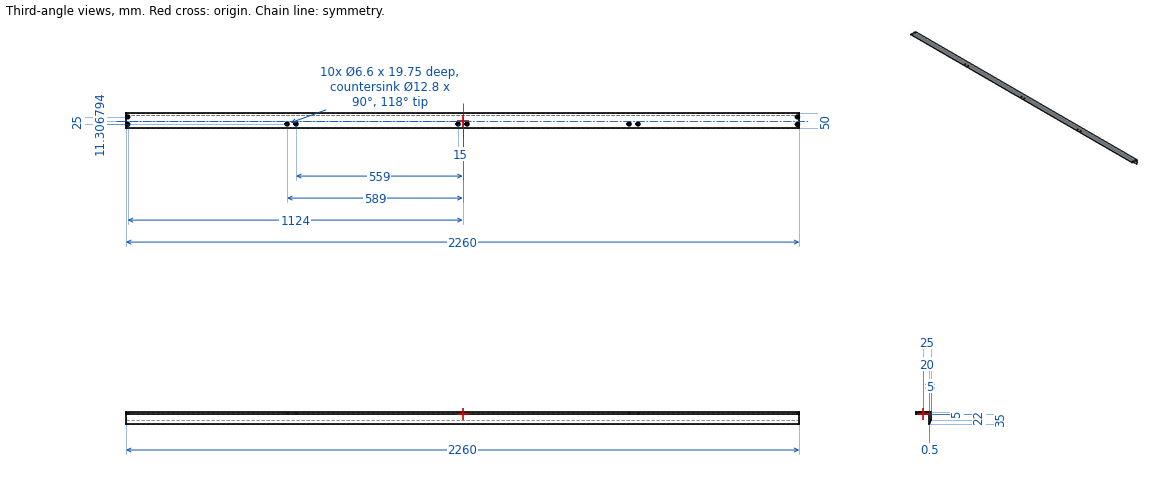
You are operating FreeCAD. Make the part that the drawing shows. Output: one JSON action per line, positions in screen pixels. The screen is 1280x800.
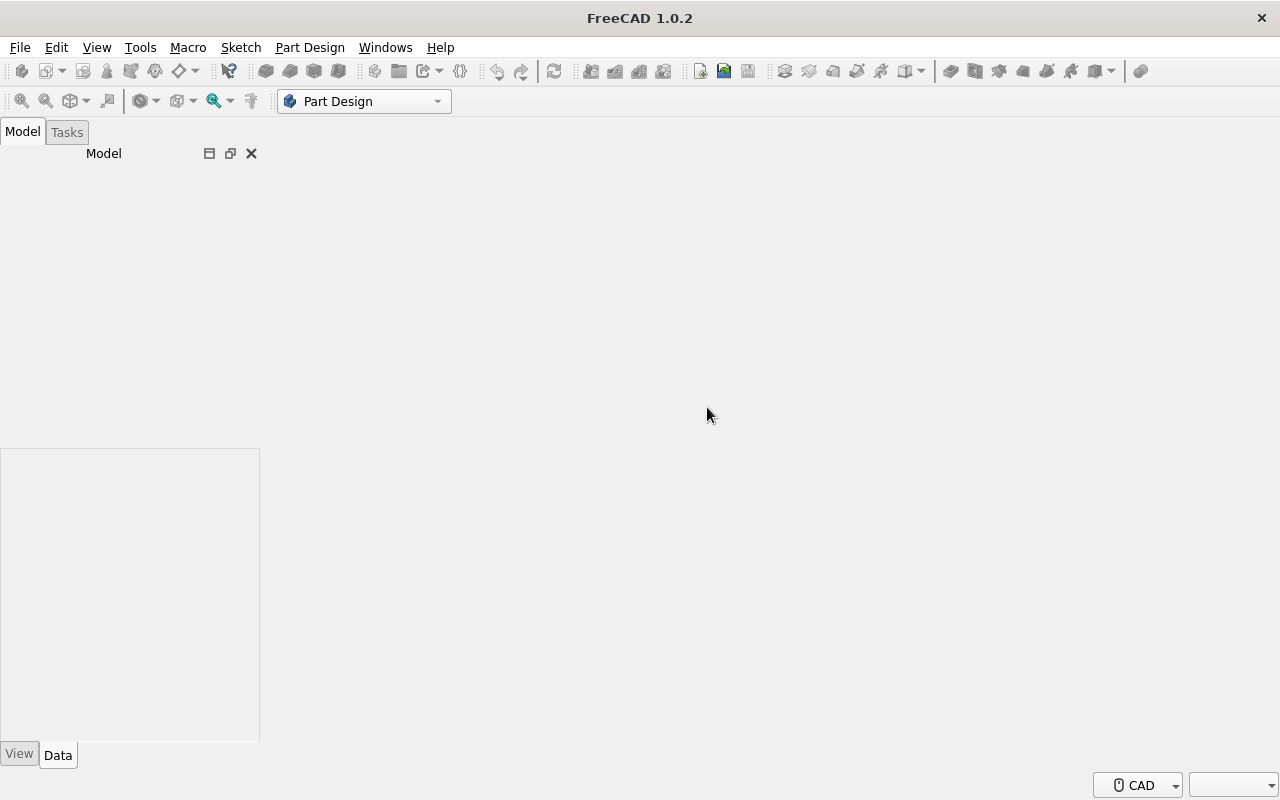
{"action": "left_click", "coordinate": [700, 72]}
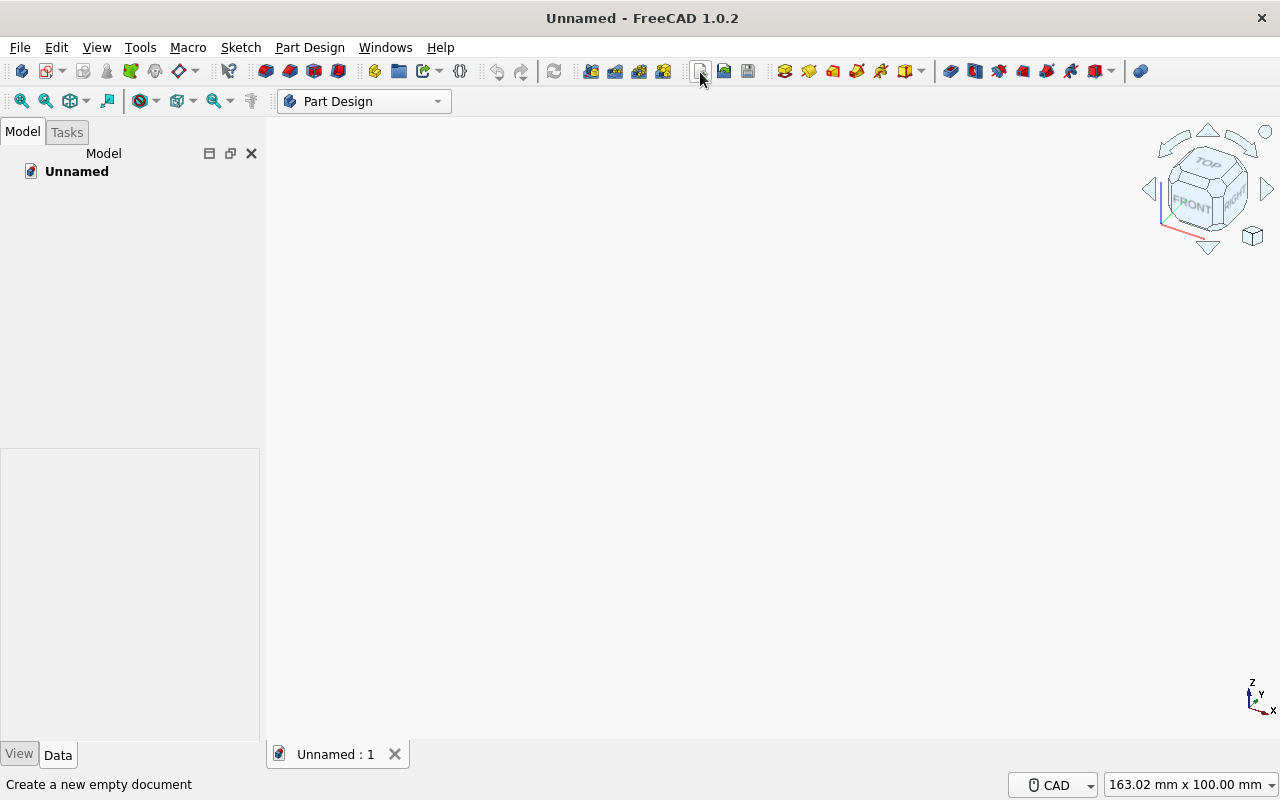
{"action": "left_click", "coordinate": [46, 72]}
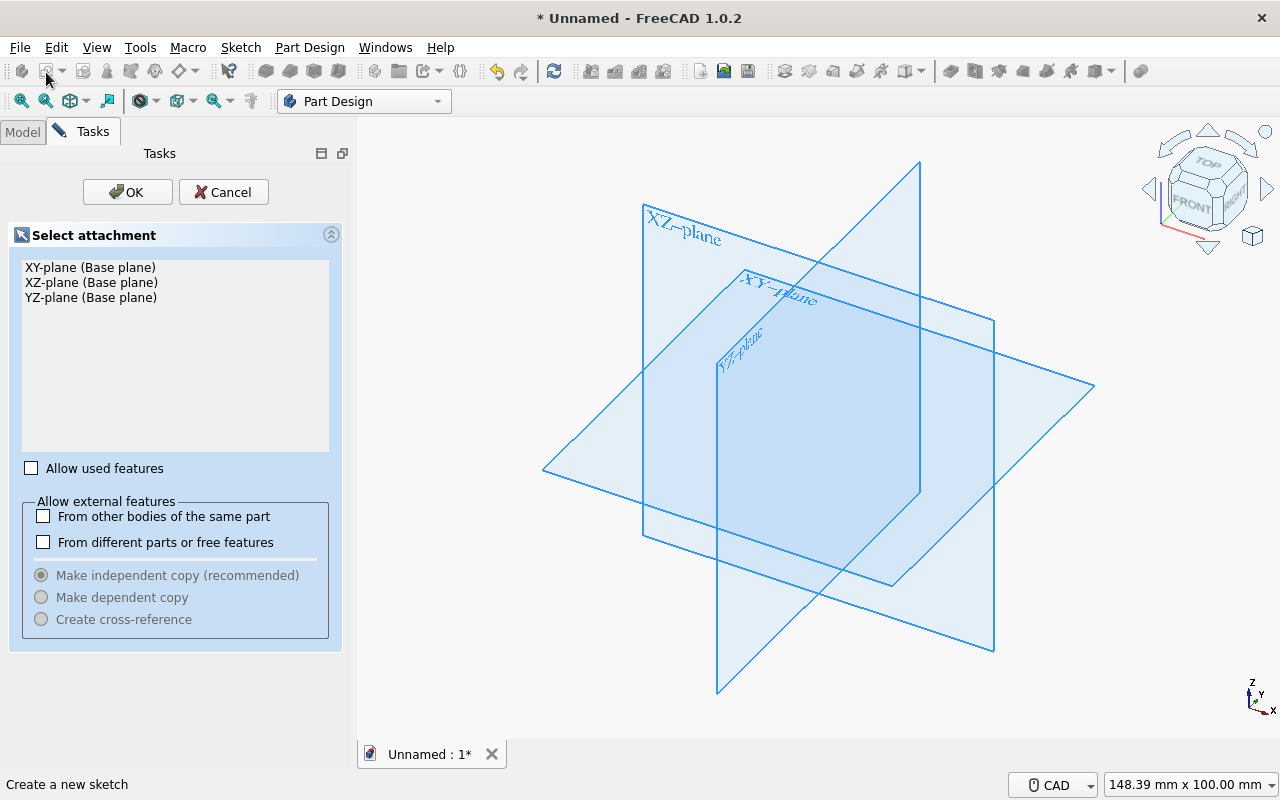
{"action": "left_click", "coordinate": [82, 268]}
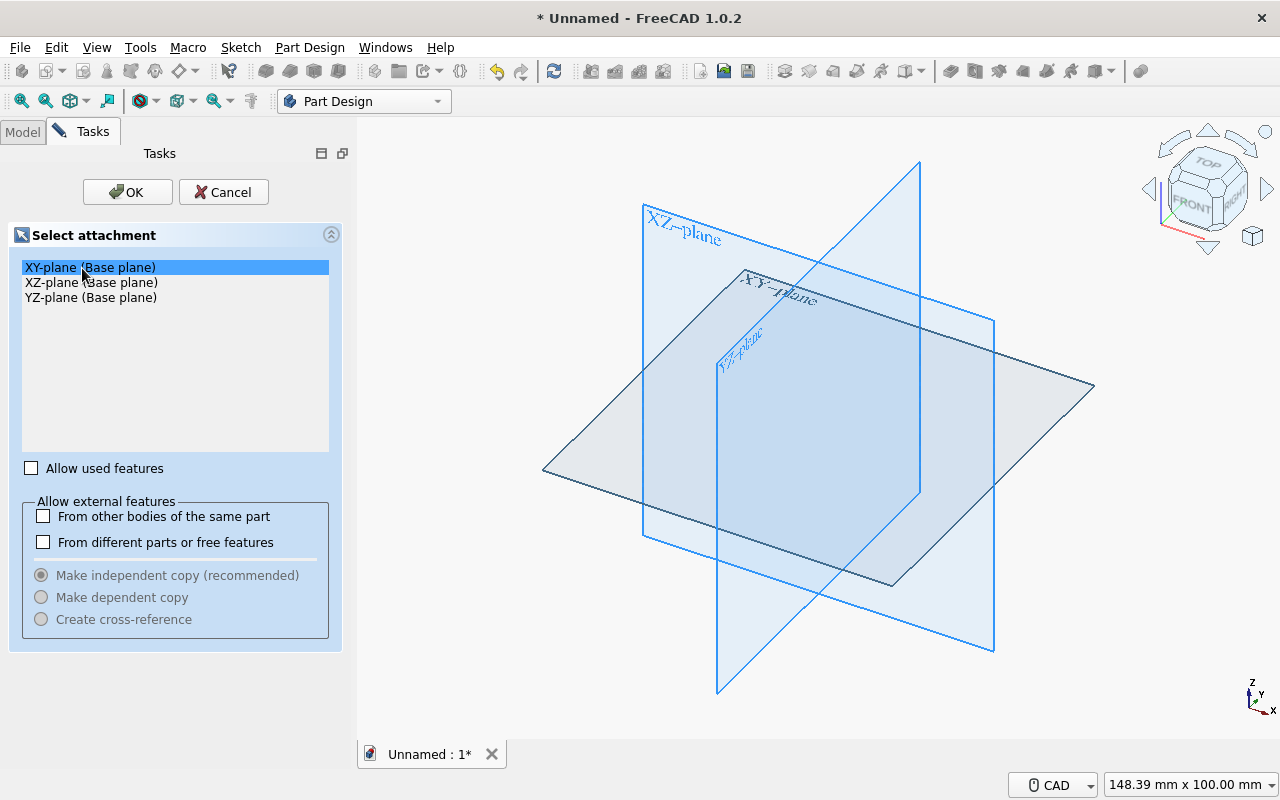
{"action": "left_click", "coordinate": [128, 192]}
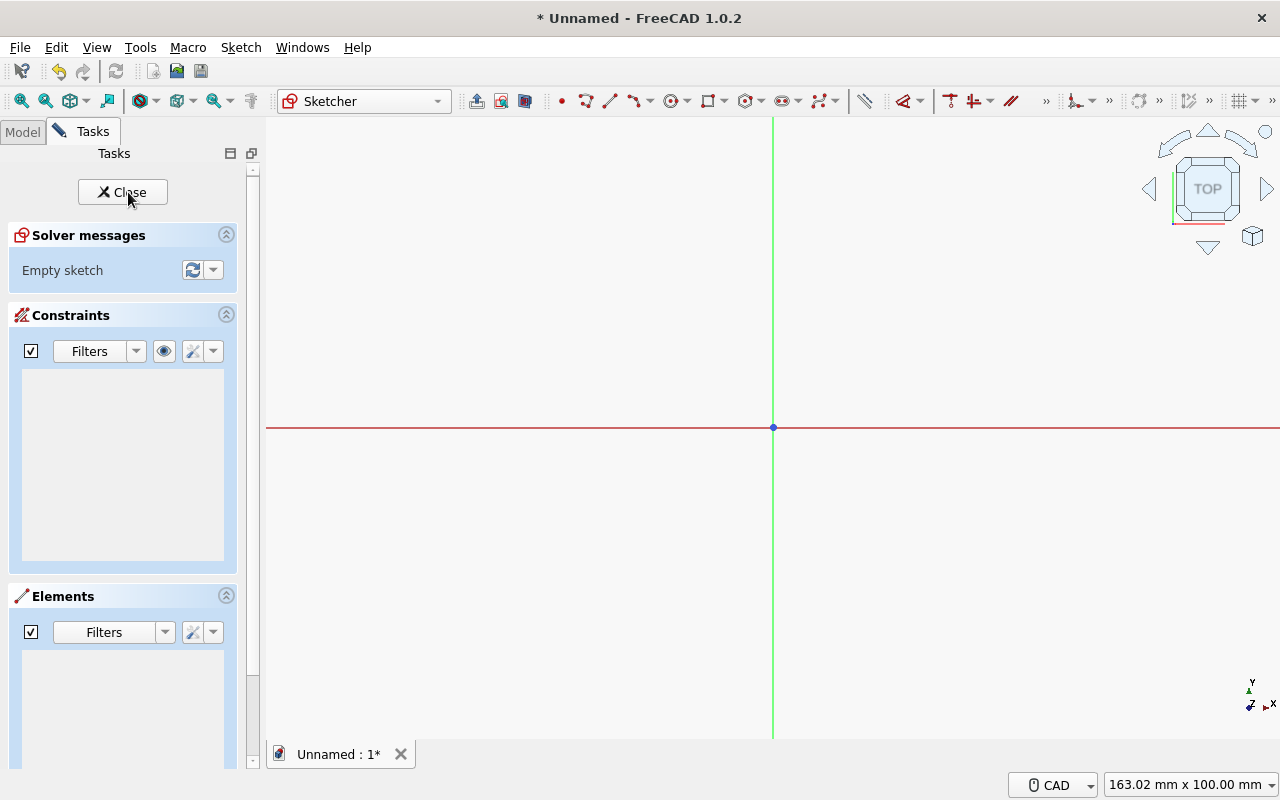
{"action": "scroll", "coordinate": [701, 428], "scroll_direction": "down", "scroll_amount": 15}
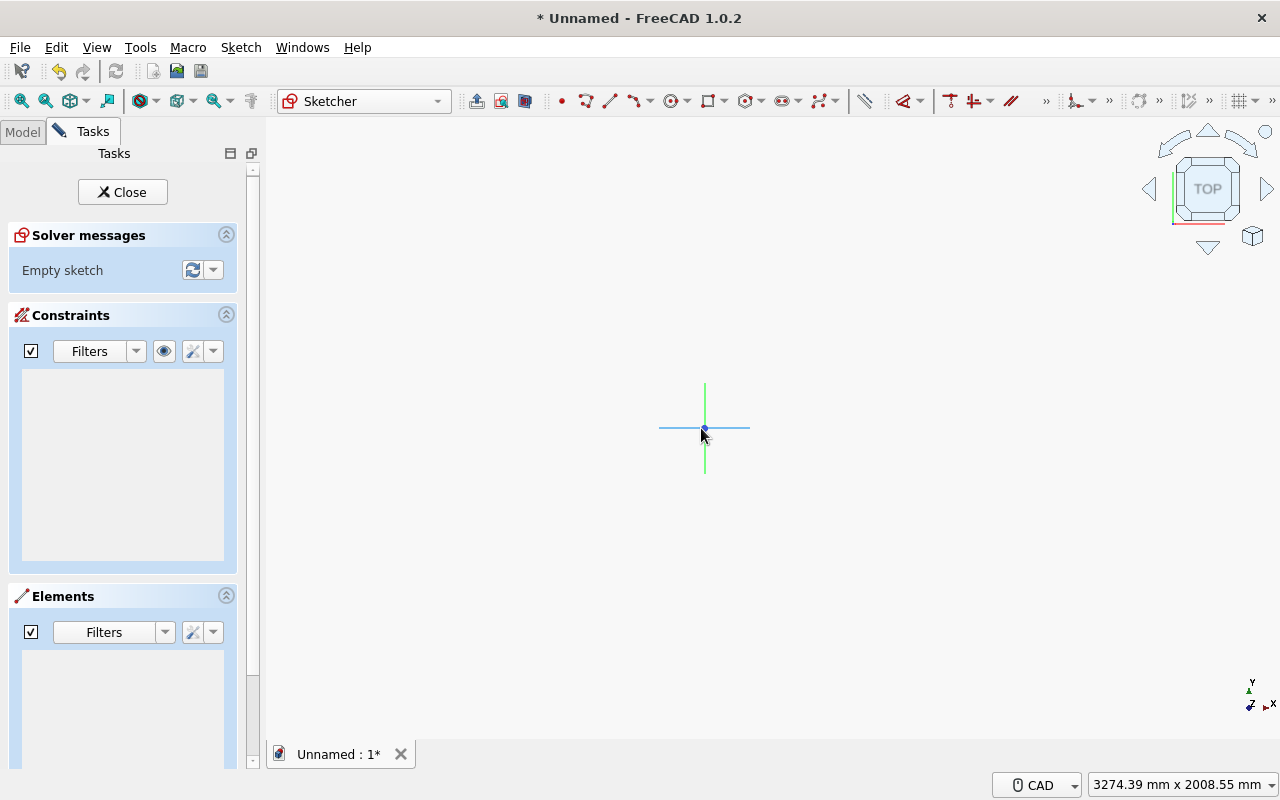
{"action": "left_click", "coordinate": [726, 102]}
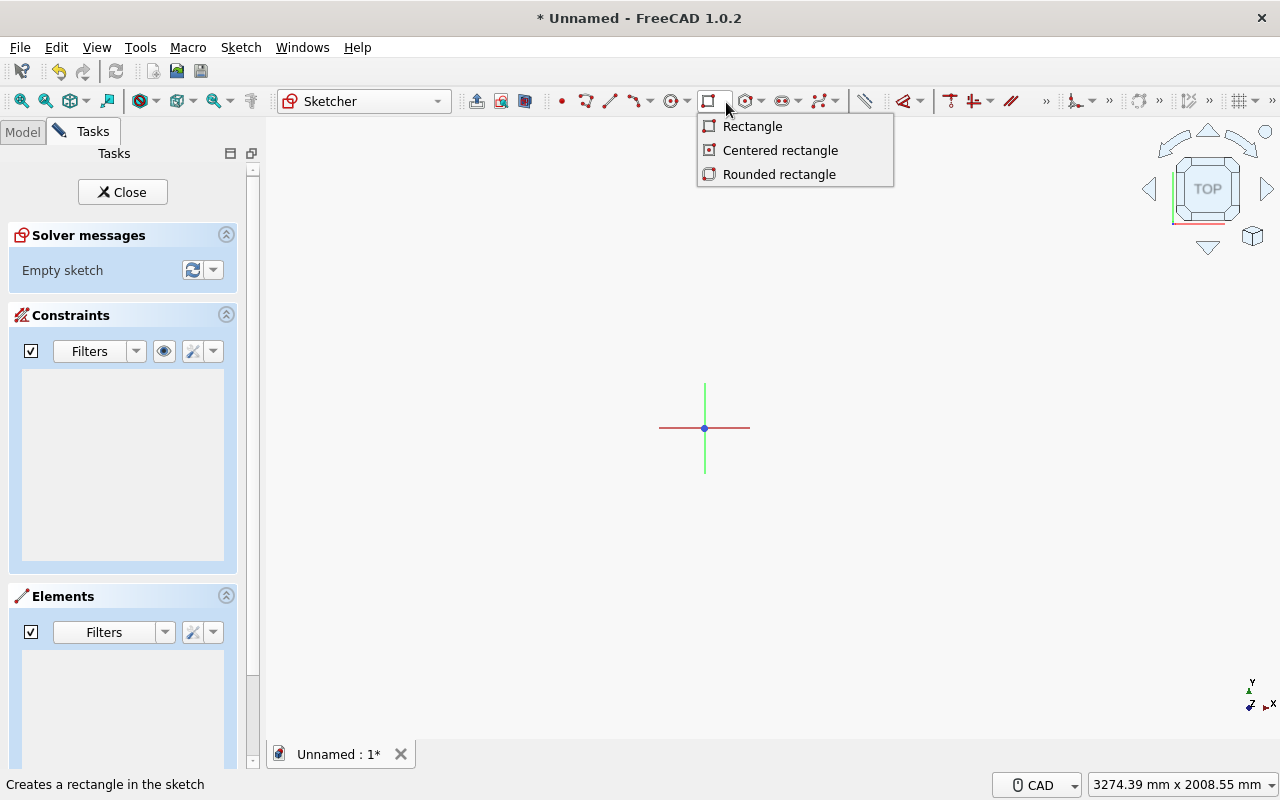
{"action": "left_click", "coordinate": [796, 150]}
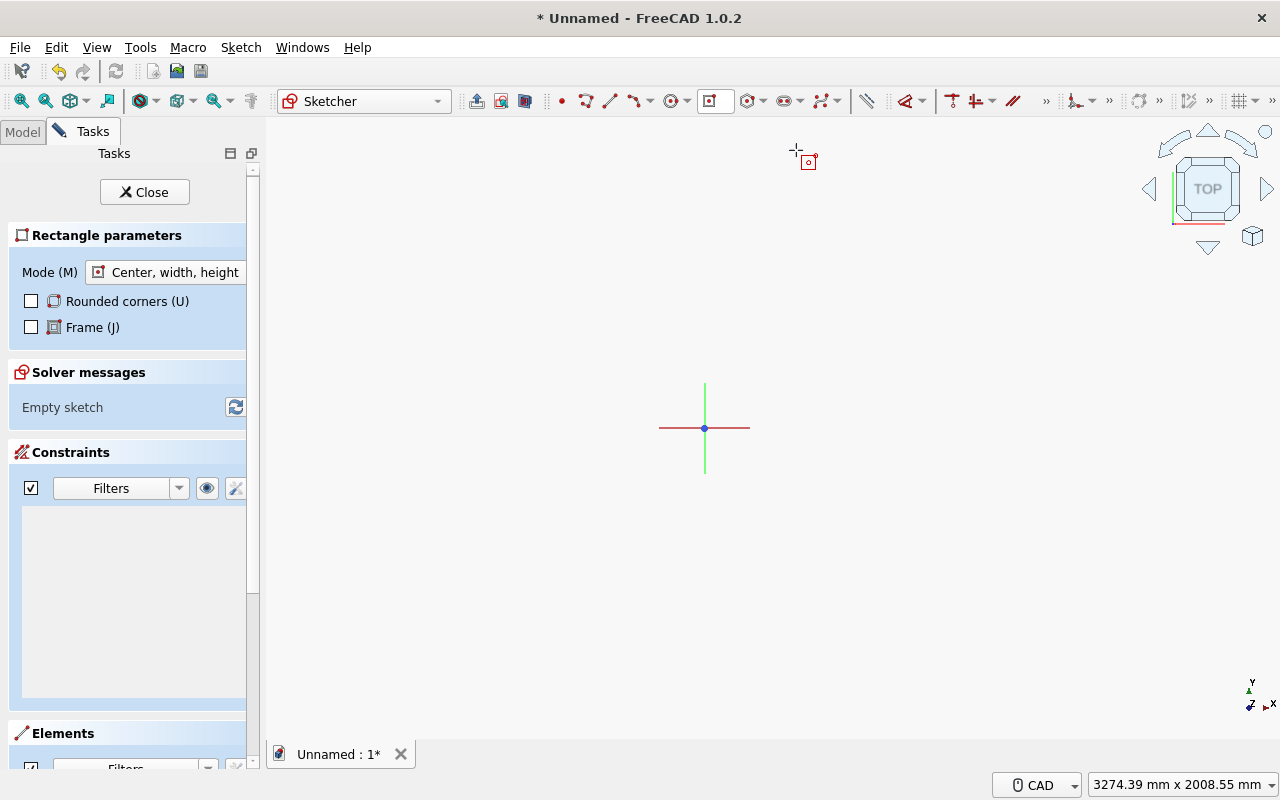
{"action": "scroll", "coordinate": [705, 428], "scroll_direction": "up", "scroll_amount": 4}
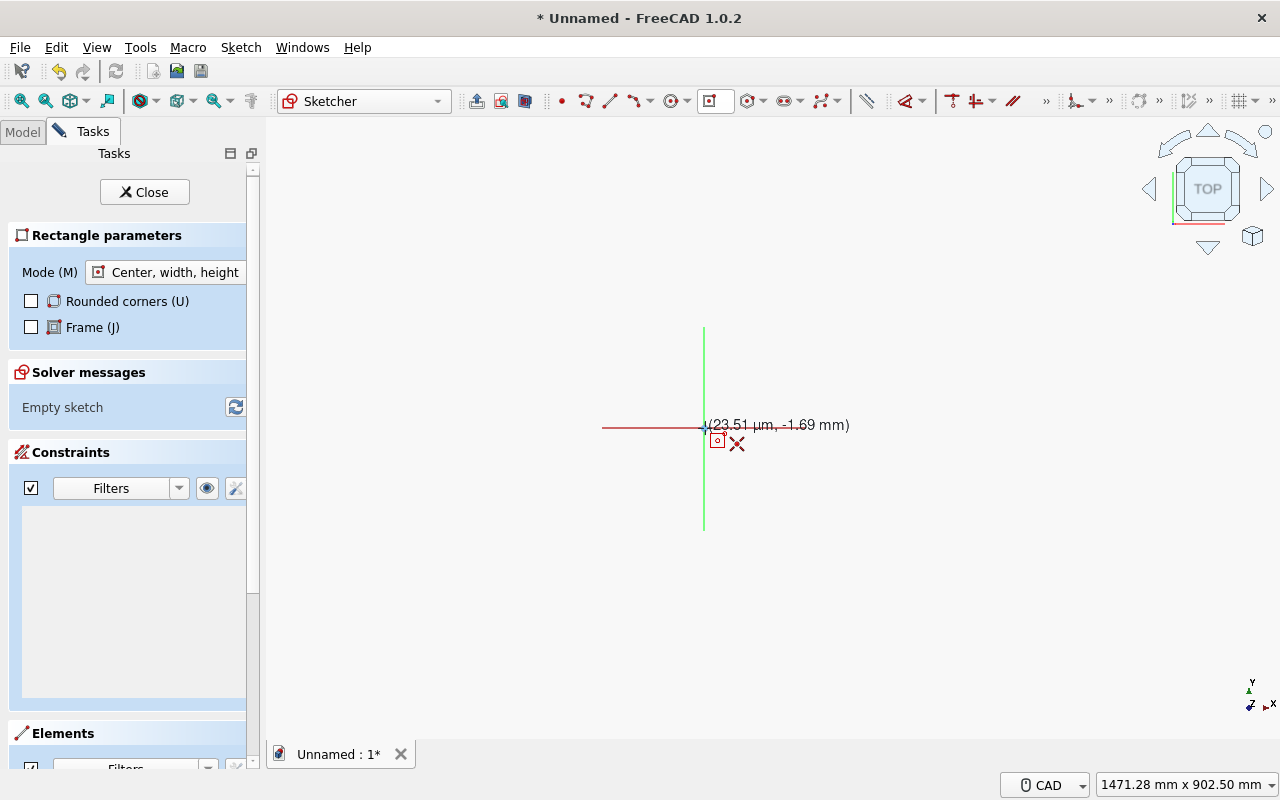
{"action": "left_click", "coordinate": [704, 428]}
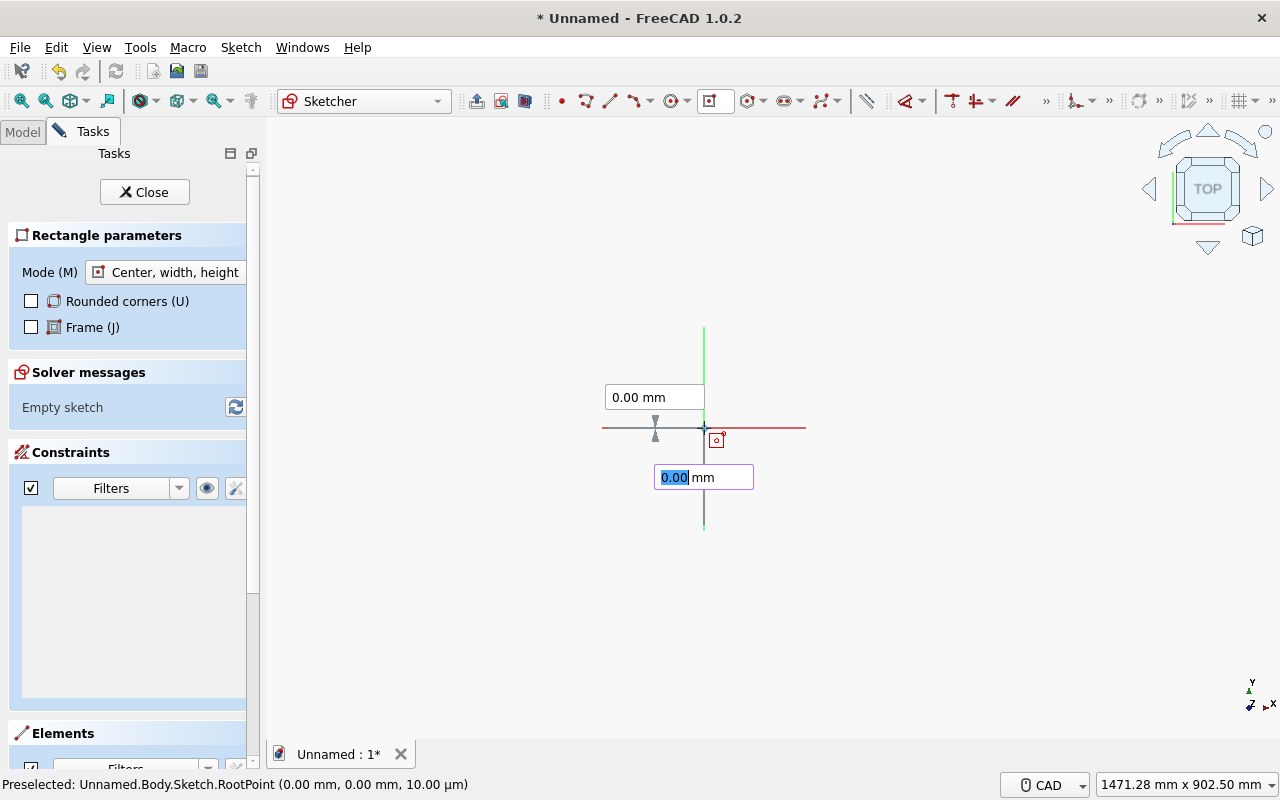
{"action": "scroll", "coordinate": [705, 428], "scroll_direction": "down", "scroll_amount": 5}